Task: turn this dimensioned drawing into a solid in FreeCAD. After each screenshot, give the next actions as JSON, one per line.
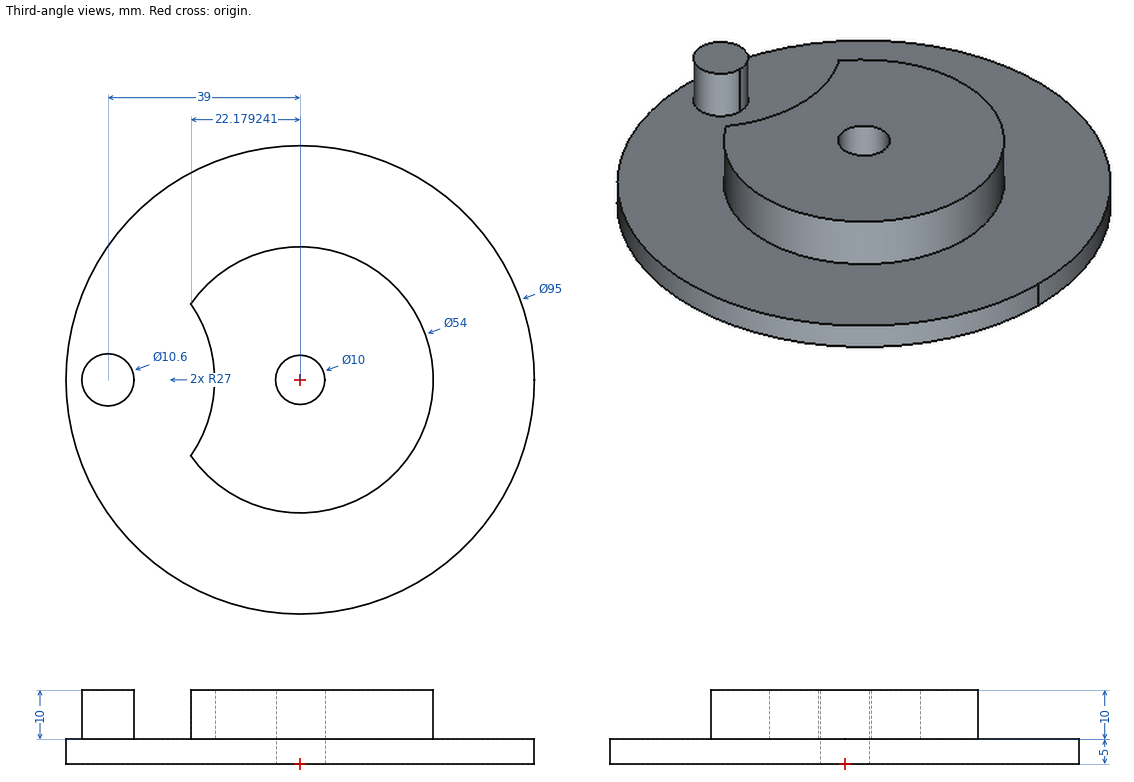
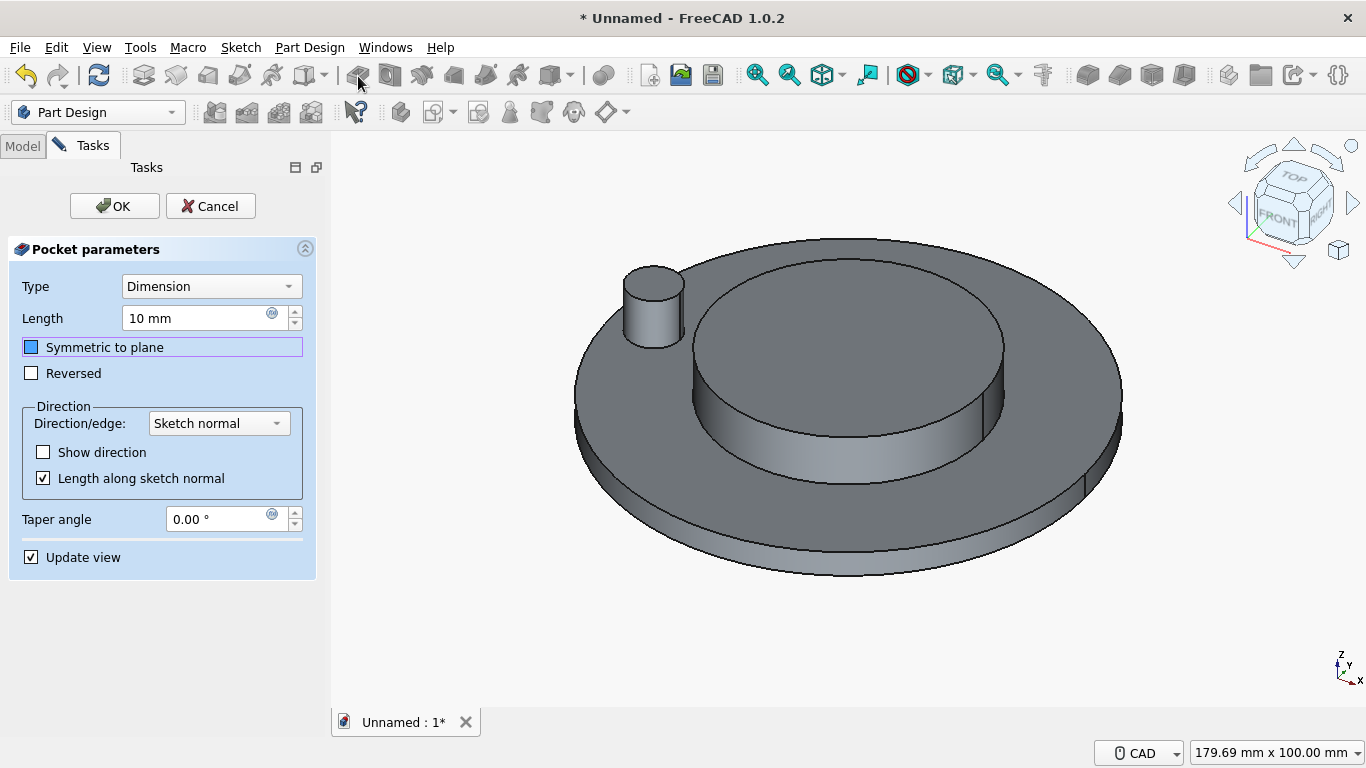
{"action": "left_click", "coordinate": [30, 373]}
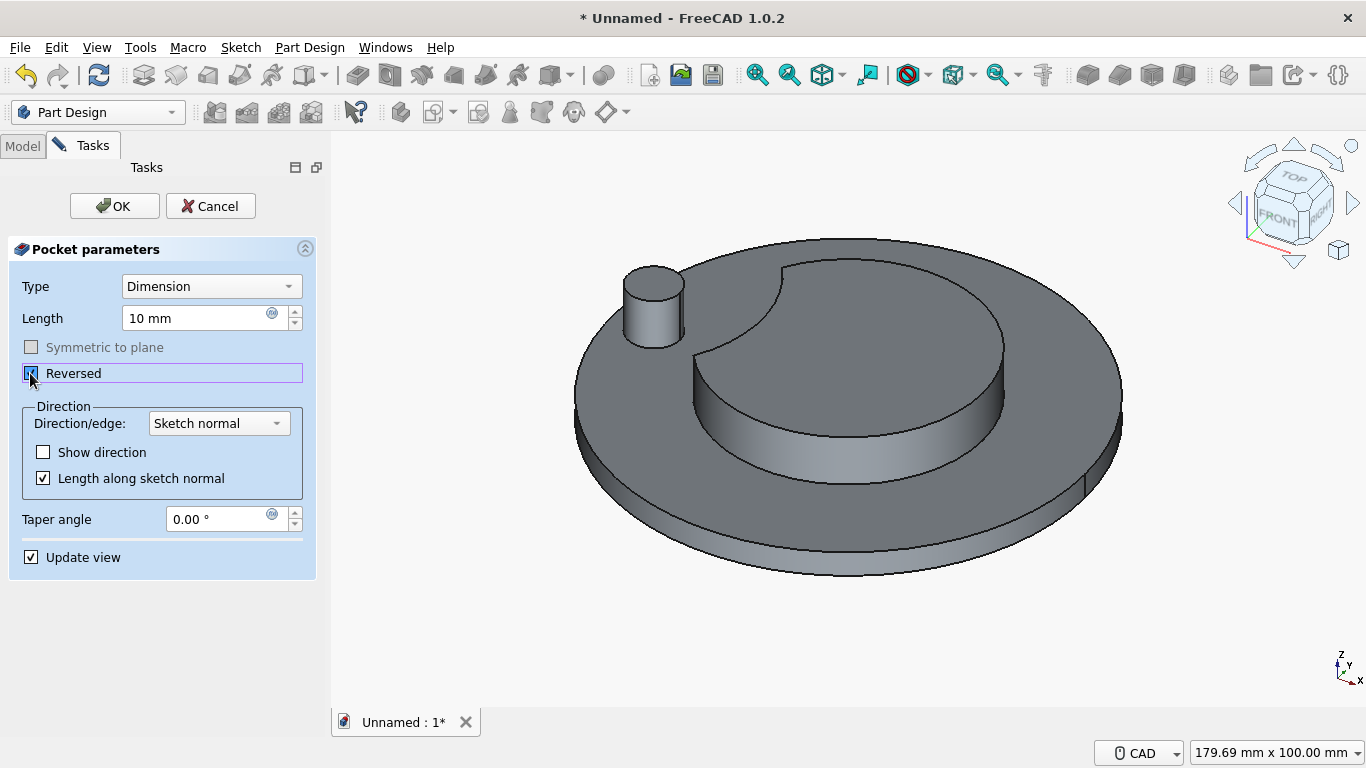
{"action": "left_click", "coordinate": [115, 206]}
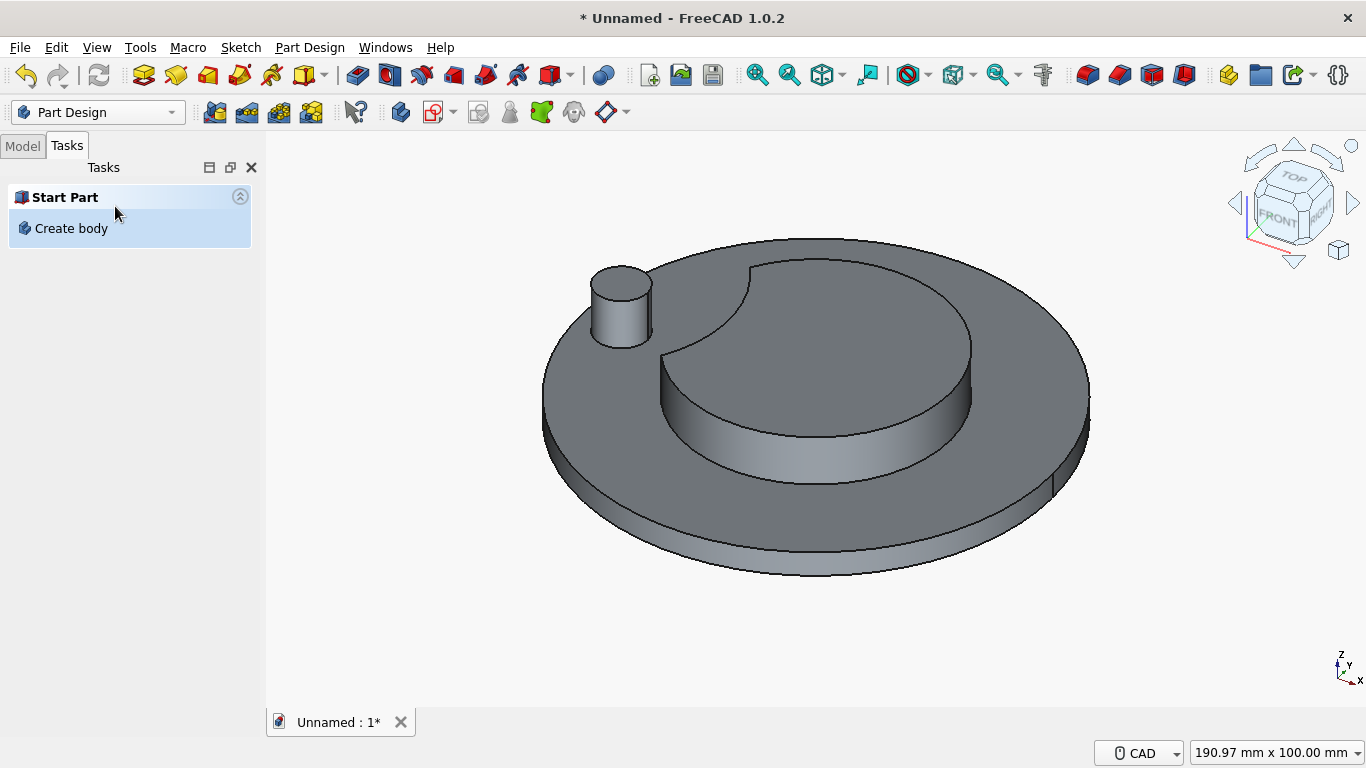
{"action": "left_click", "coordinate": [828, 351]}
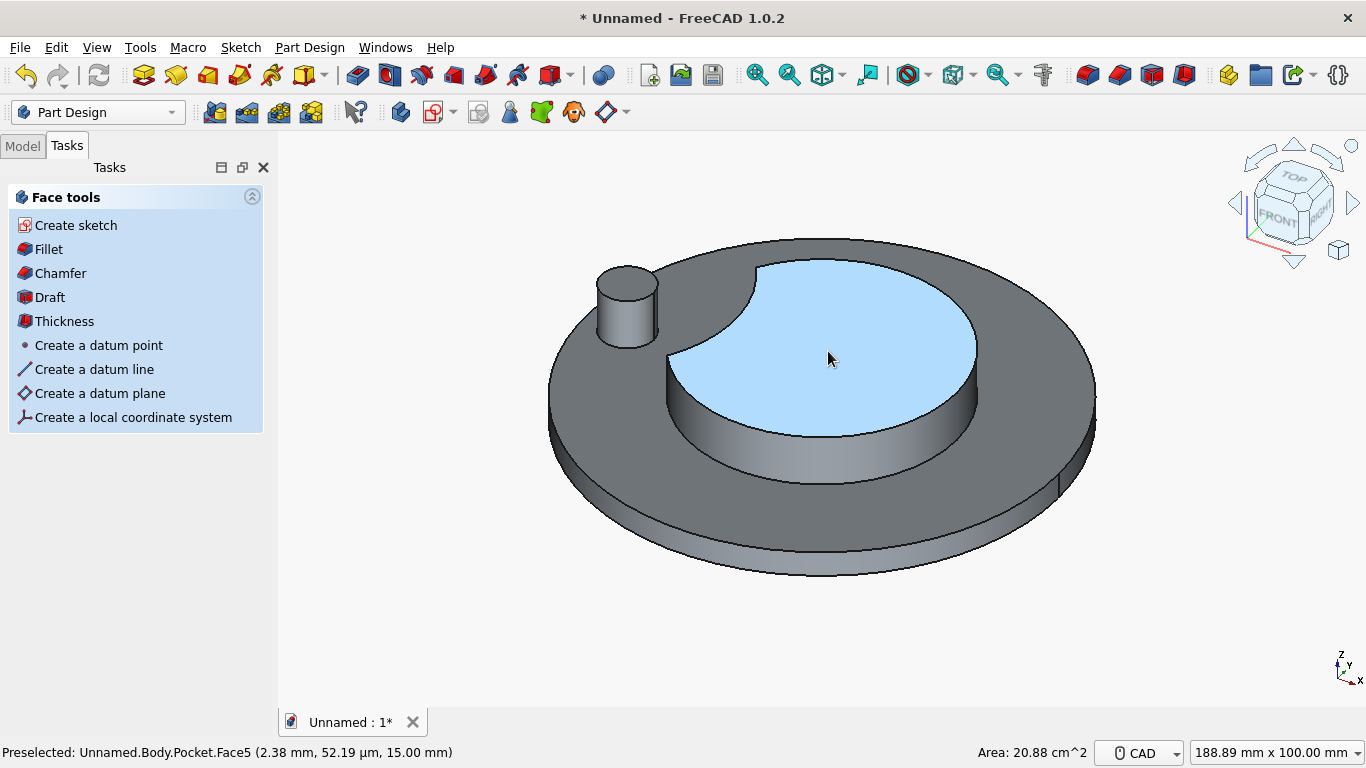
{"action": "left_click", "coordinate": [434, 112]}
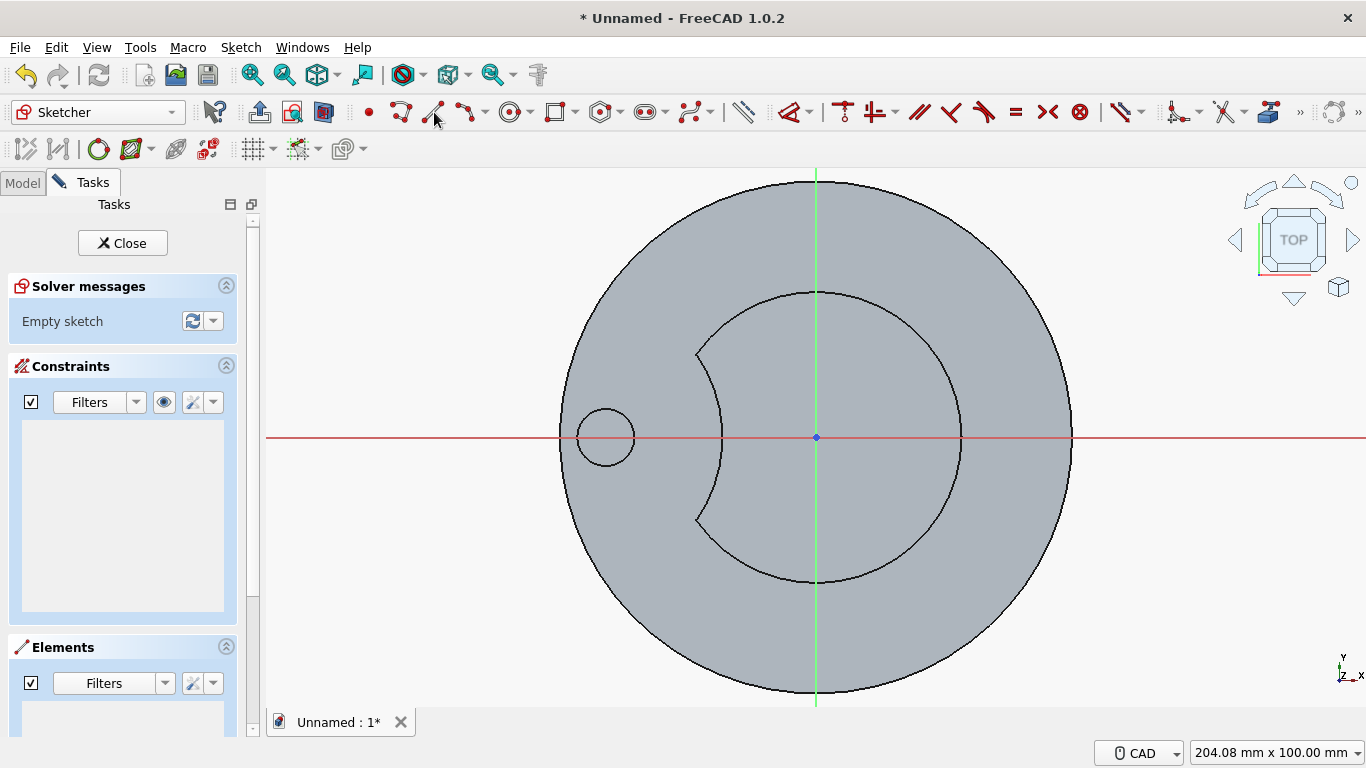
{"action": "scroll", "coordinate": [830, 438], "scroll_direction": "up", "scroll_amount": 9}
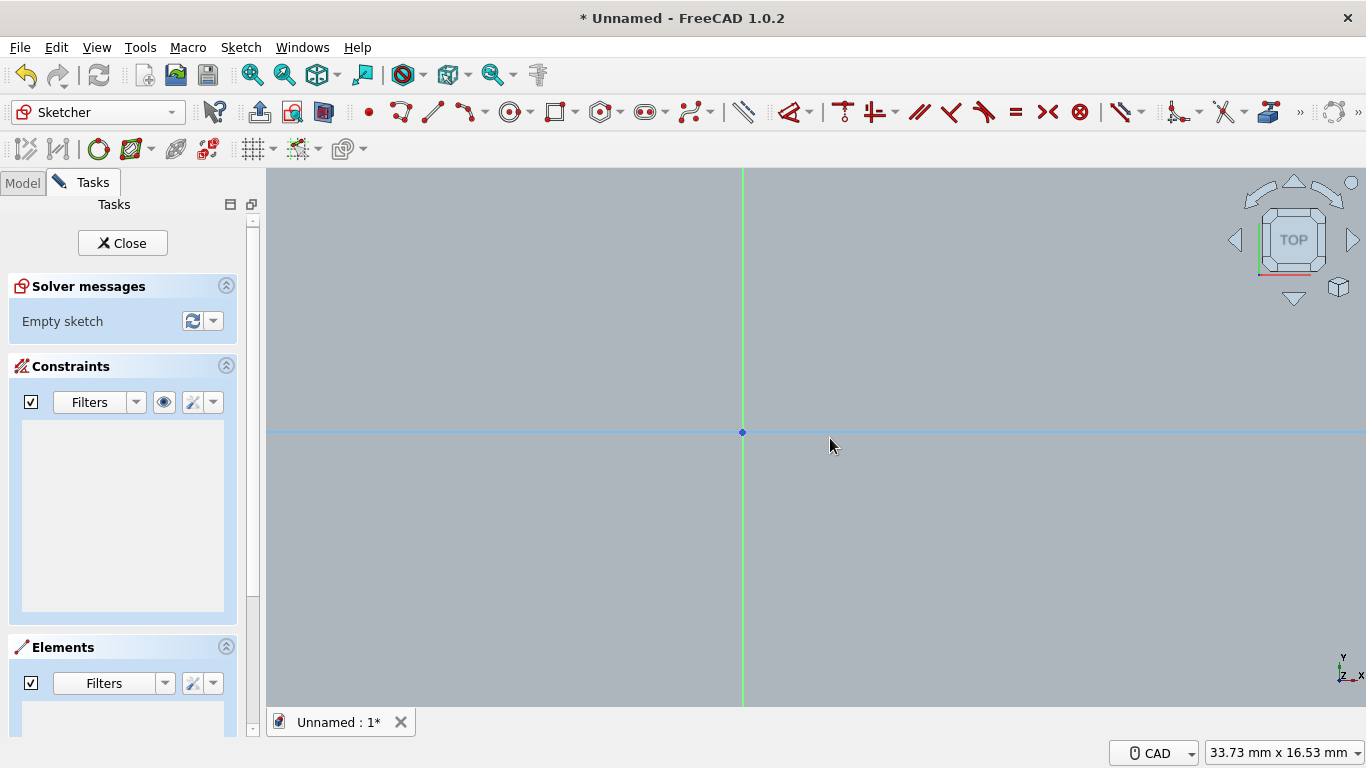
{"action": "key", "text": "g c"}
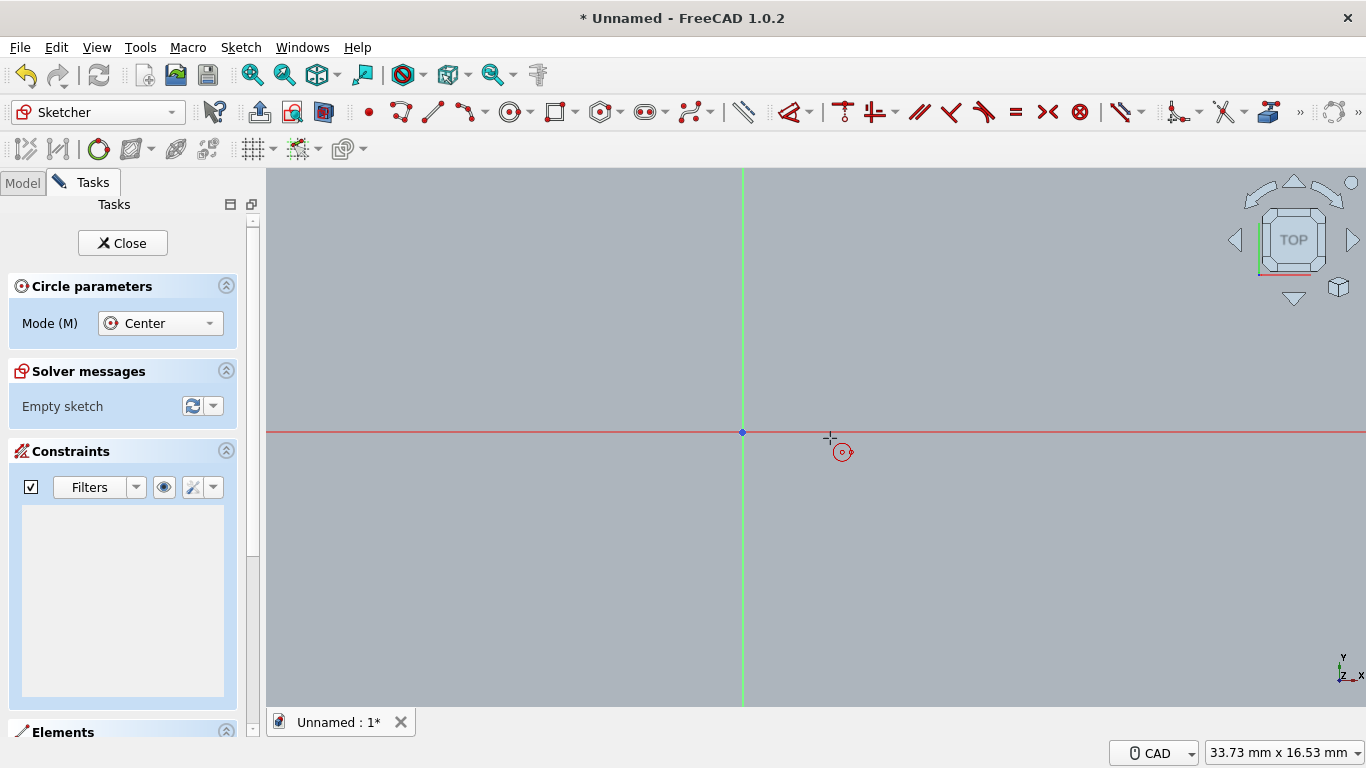
{"action": "left_click", "coordinate": [743, 432]}
{"action": "left_click", "coordinate": [858, 317]}
{"action": "key", "text": "Escape"}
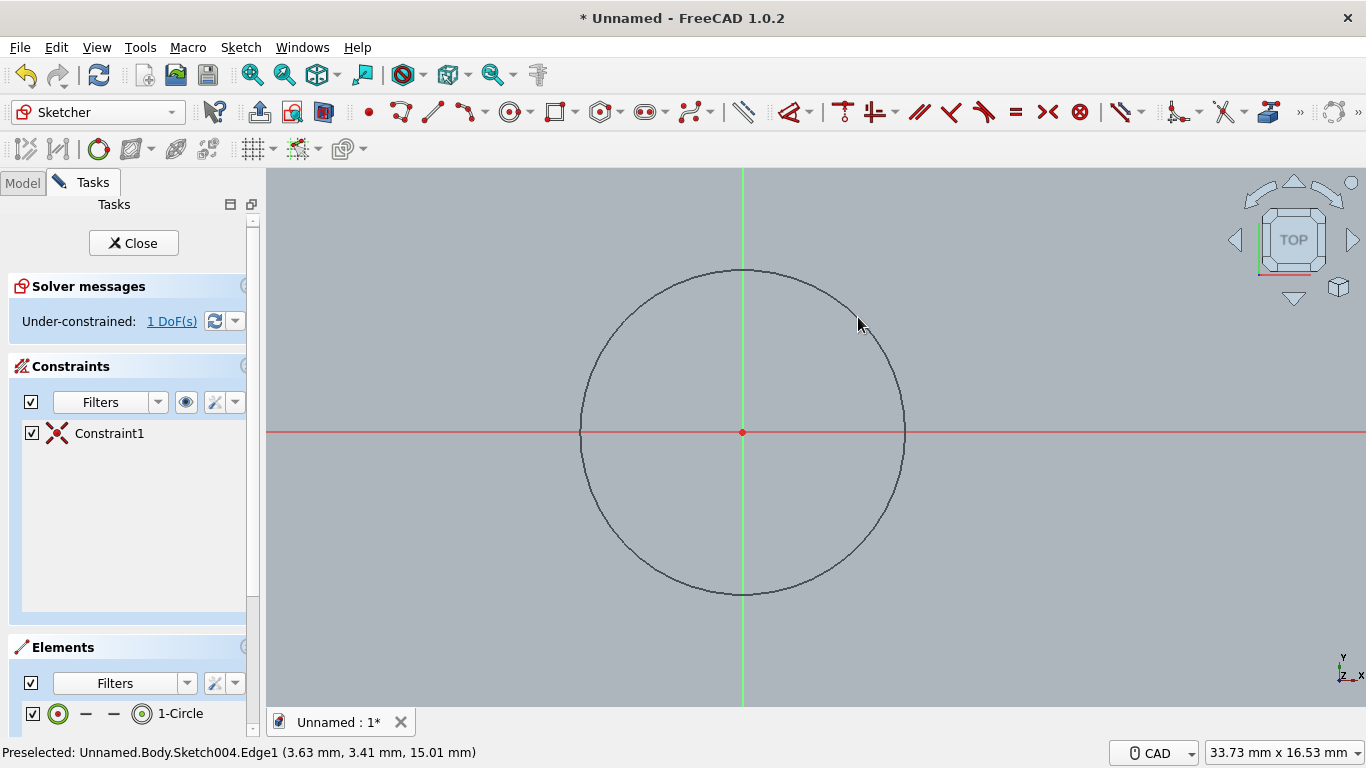
{"action": "key", "text": "d"}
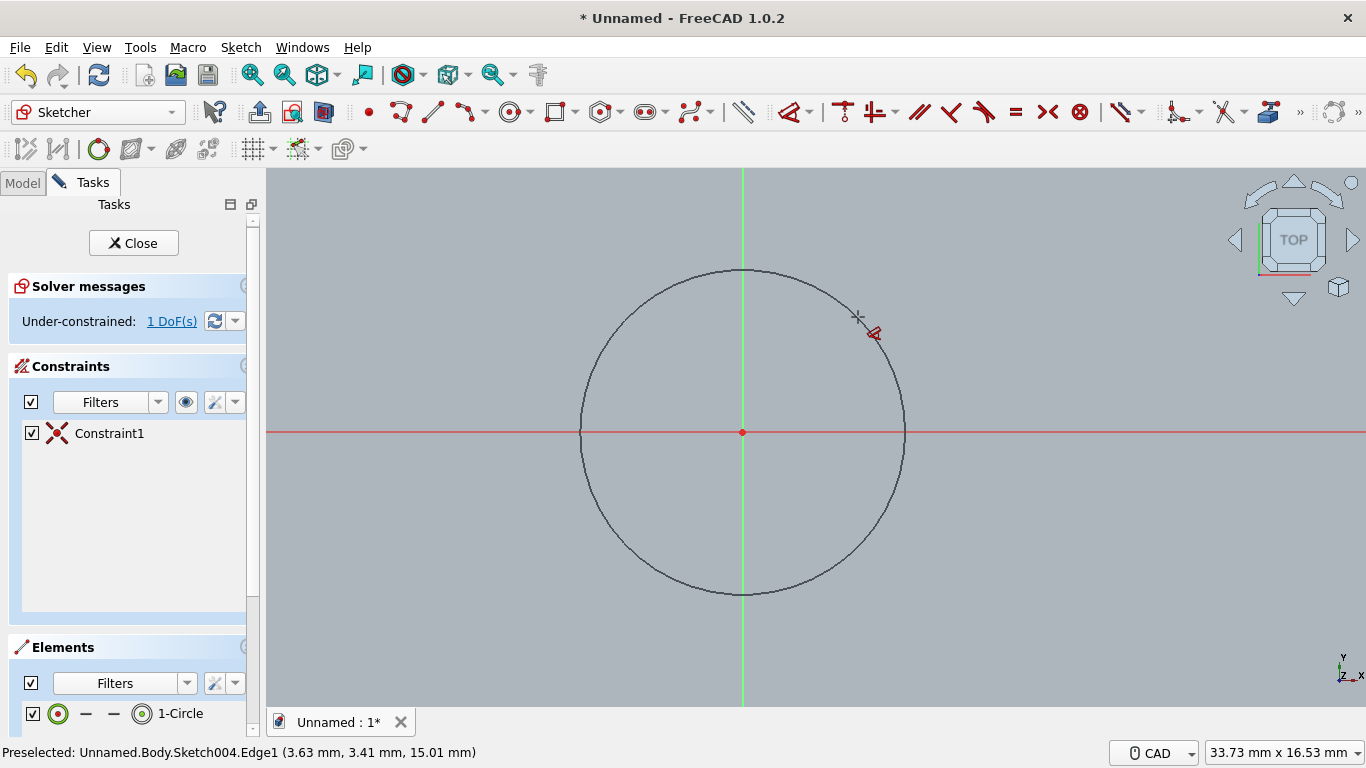
{"action": "left_click", "coordinate": [857, 317]}
{"action": "left_click", "coordinate": [880, 294]}